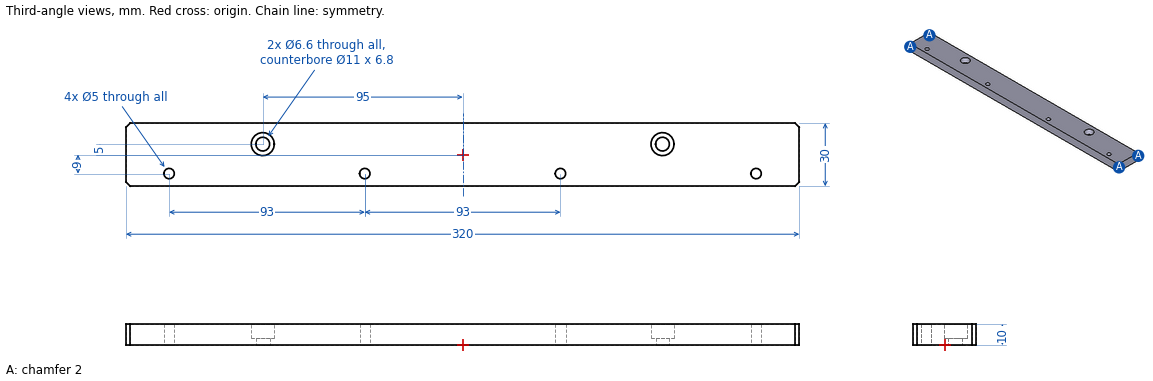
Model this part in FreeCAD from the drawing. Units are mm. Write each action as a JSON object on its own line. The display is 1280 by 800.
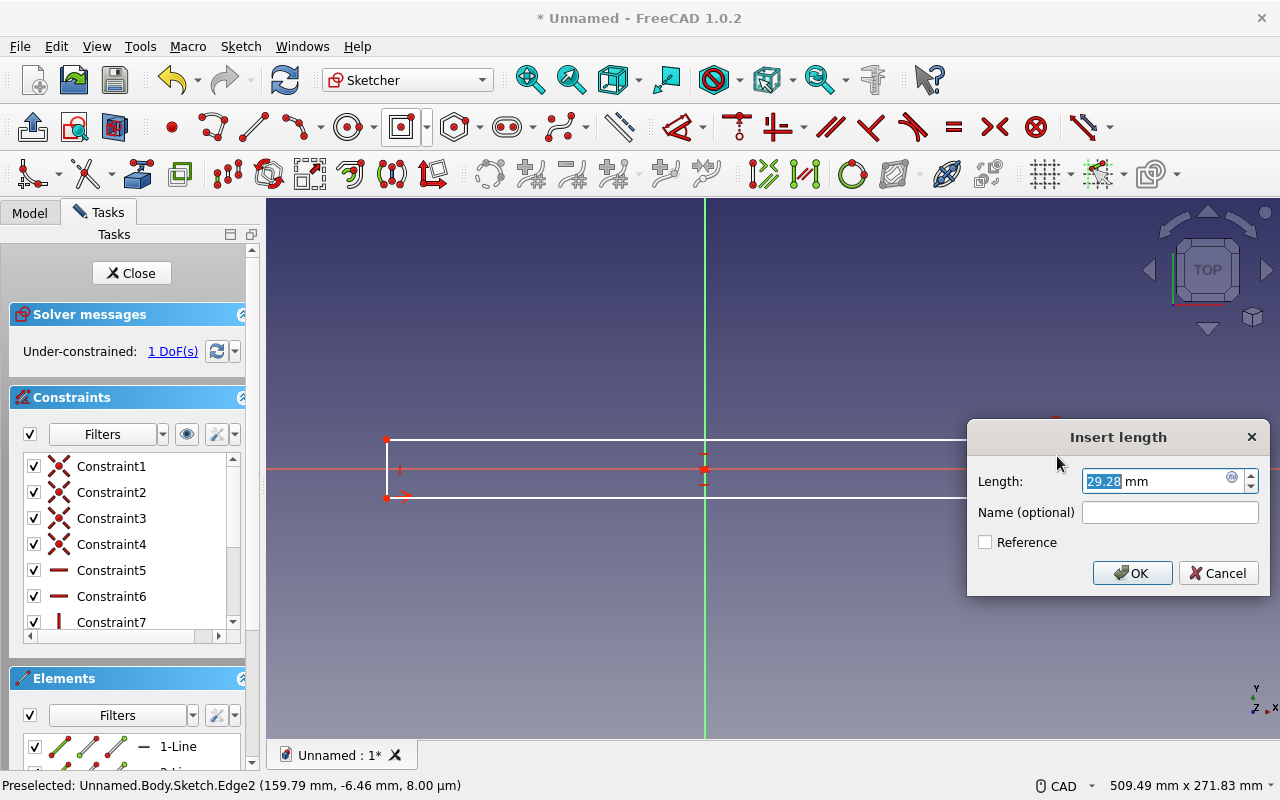
{"action": "type", "text": "30"}
{"action": "key", "text": "Return"}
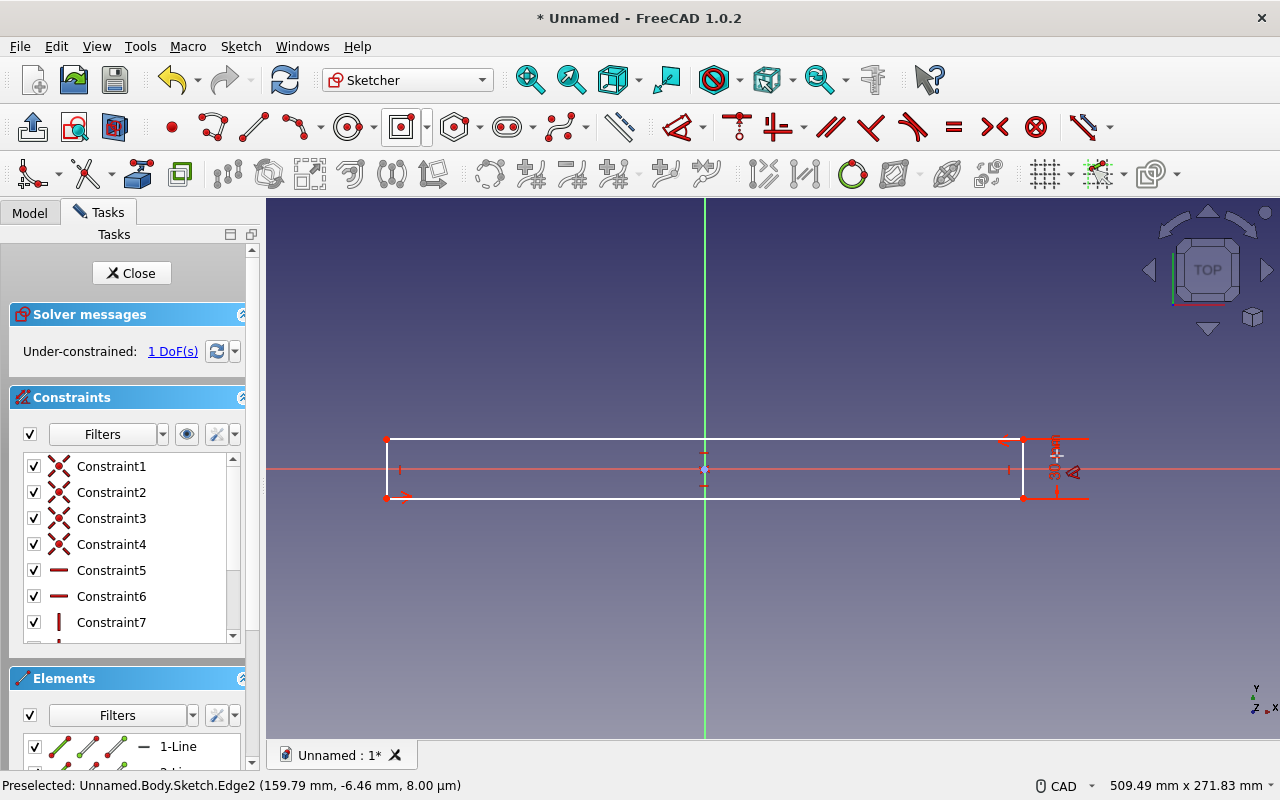
{"action": "left_click", "coordinate": [578, 499]}
{"action": "left_click", "coordinate": [559, 533]}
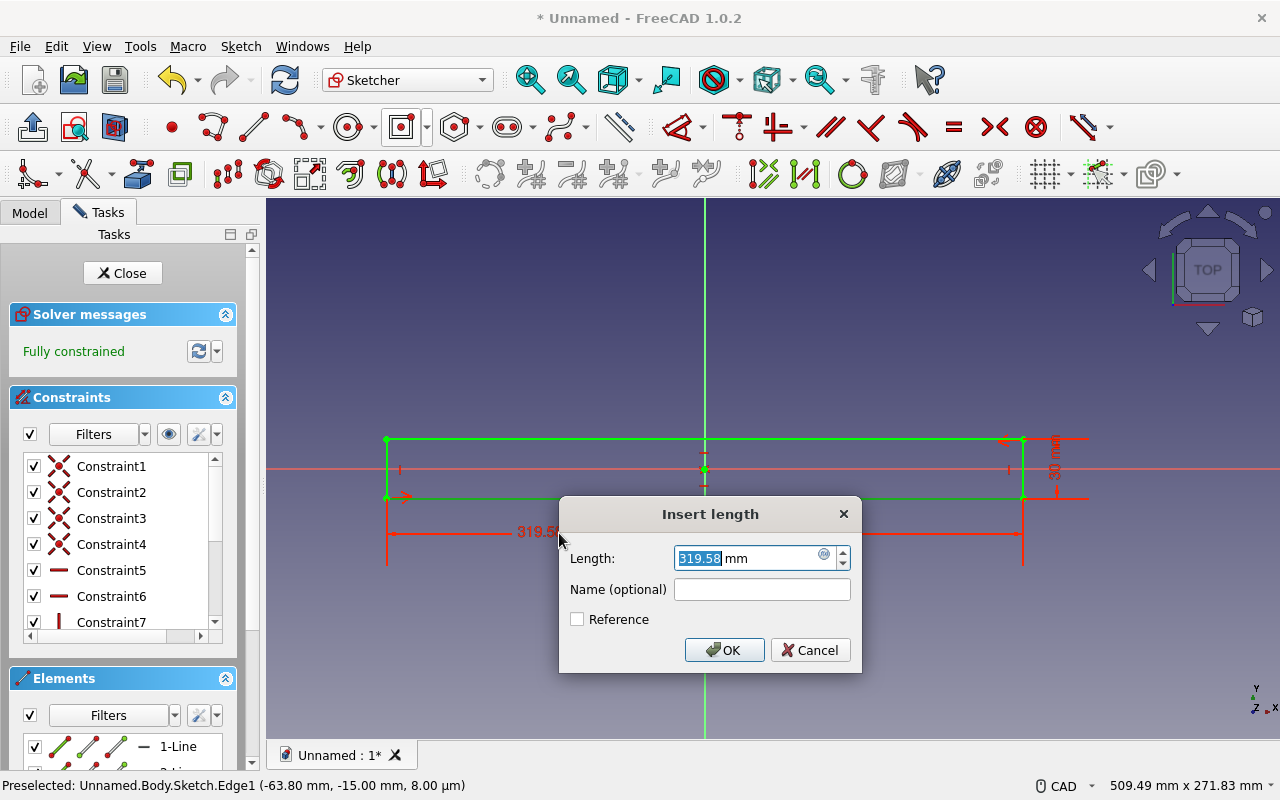
{"action": "type", "text": "320"}
{"action": "key", "text": "Return"}
{"action": "key", "text": "Escape"}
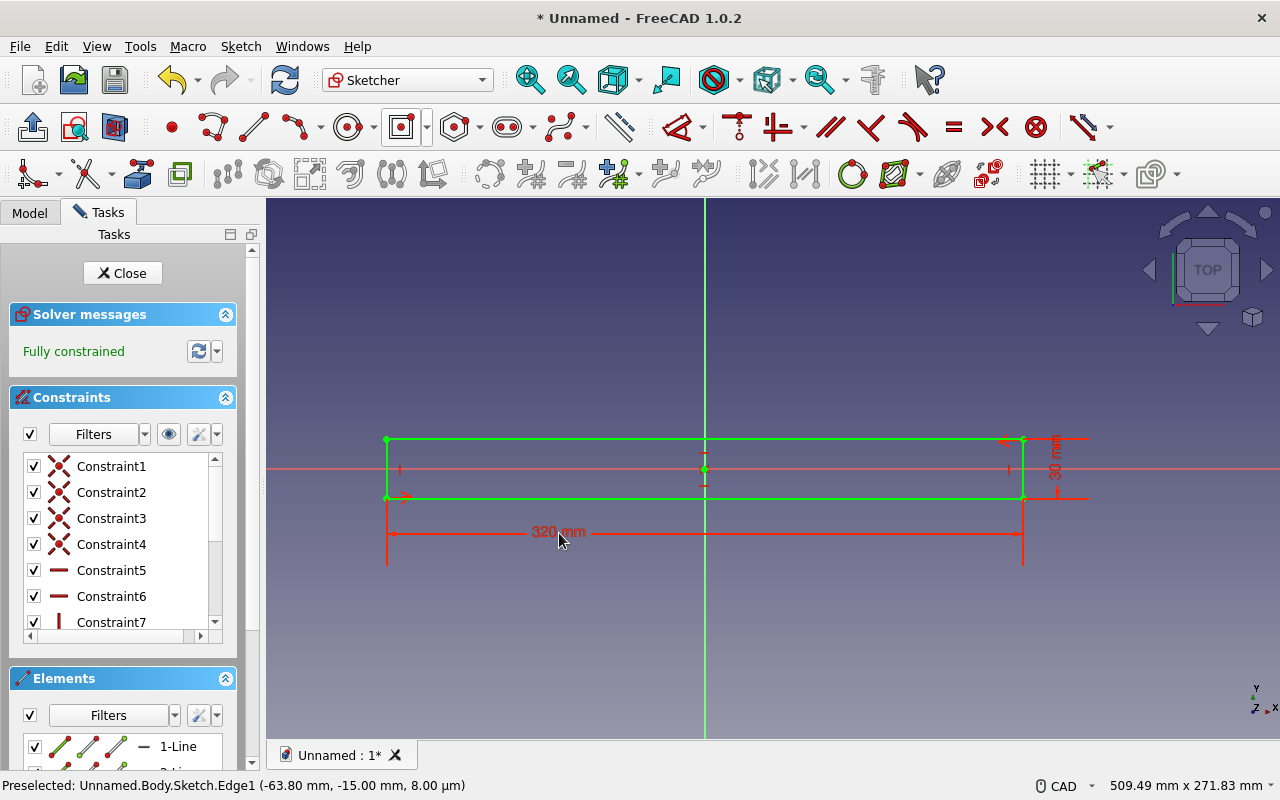
{"action": "left_click", "coordinate": [123, 273]}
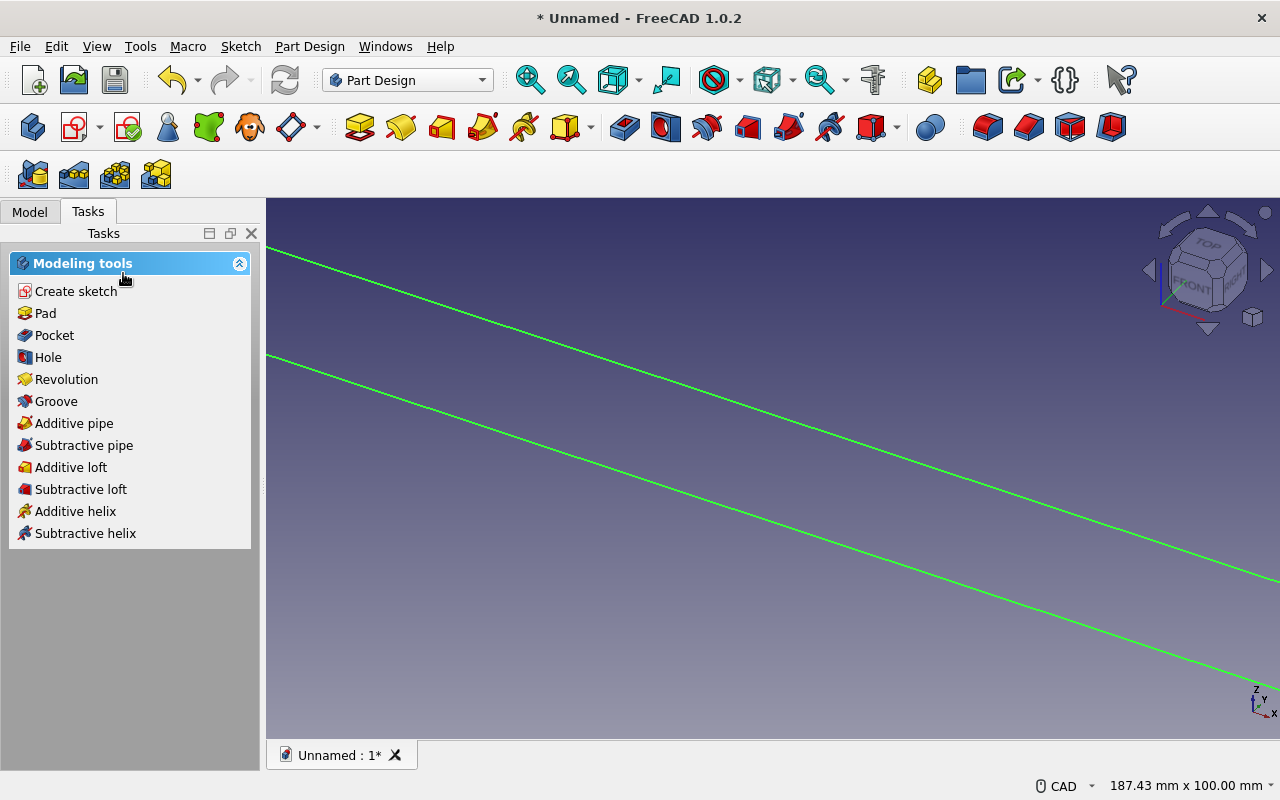
{"action": "left_click", "coordinate": [360, 128]}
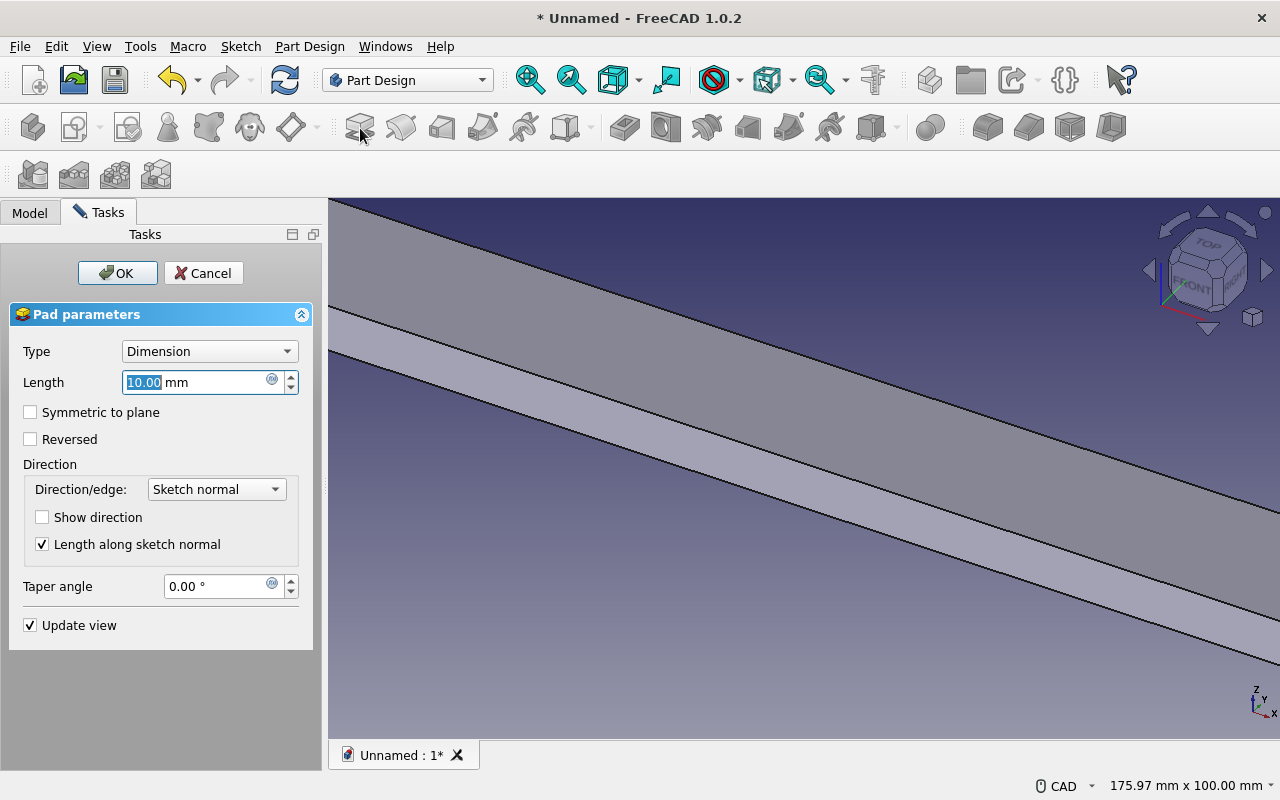
{"action": "type", "text": "10"}
{"action": "key", "text": "Tab"}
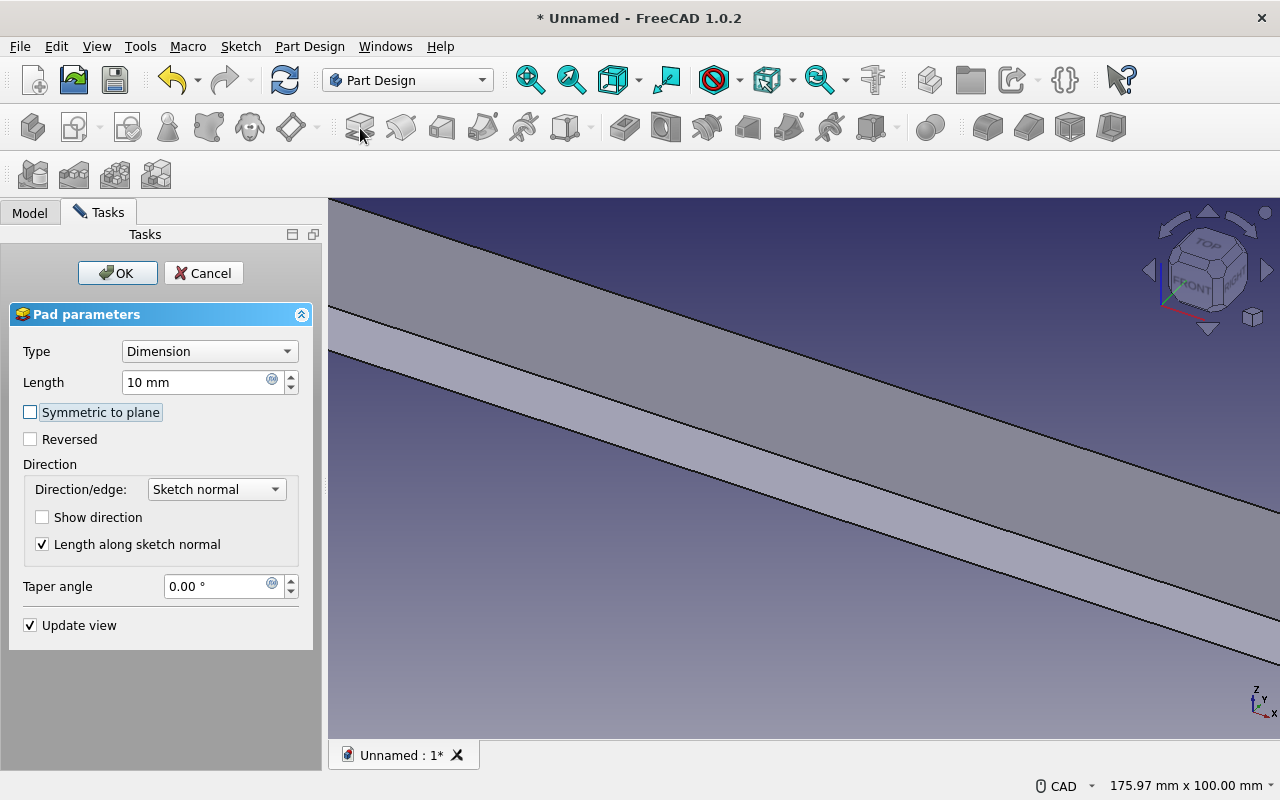
{"action": "left_click", "coordinate": [118, 273]}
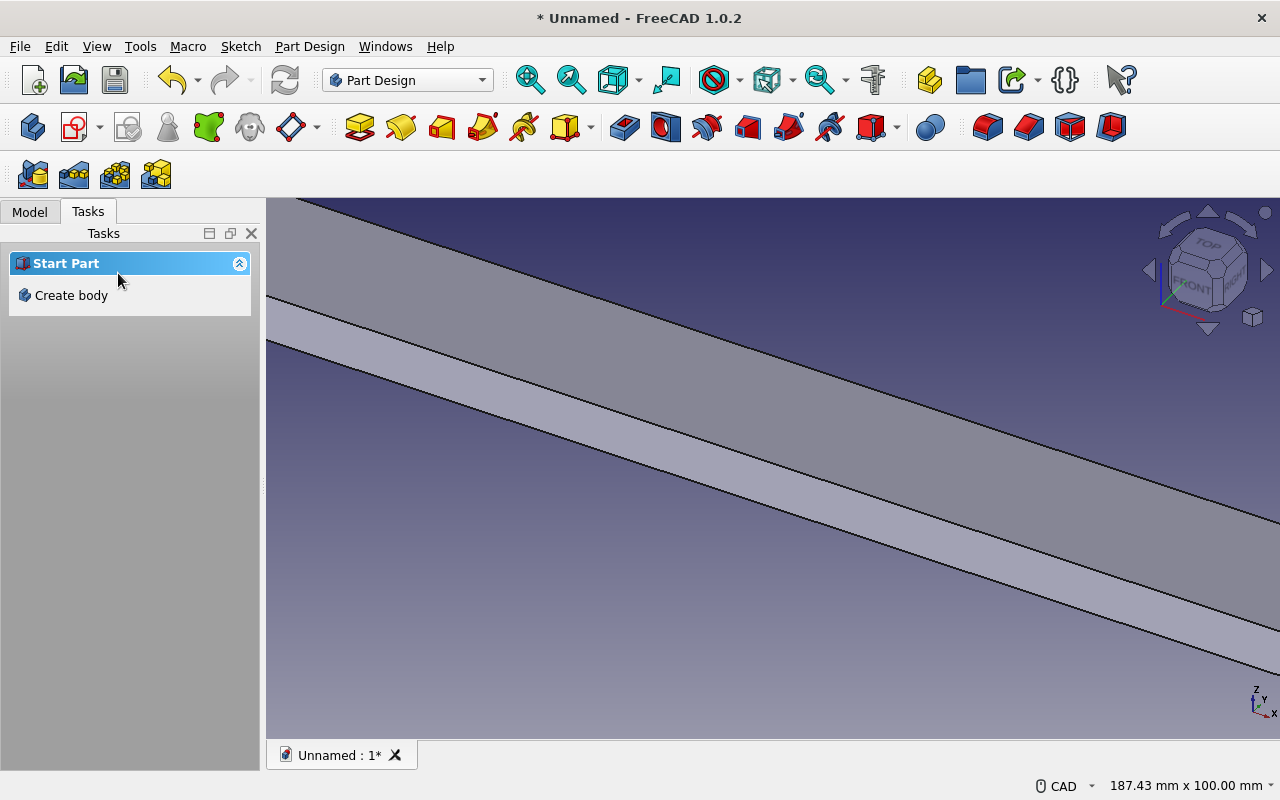
{"action": "left_click", "coordinate": [531, 80]}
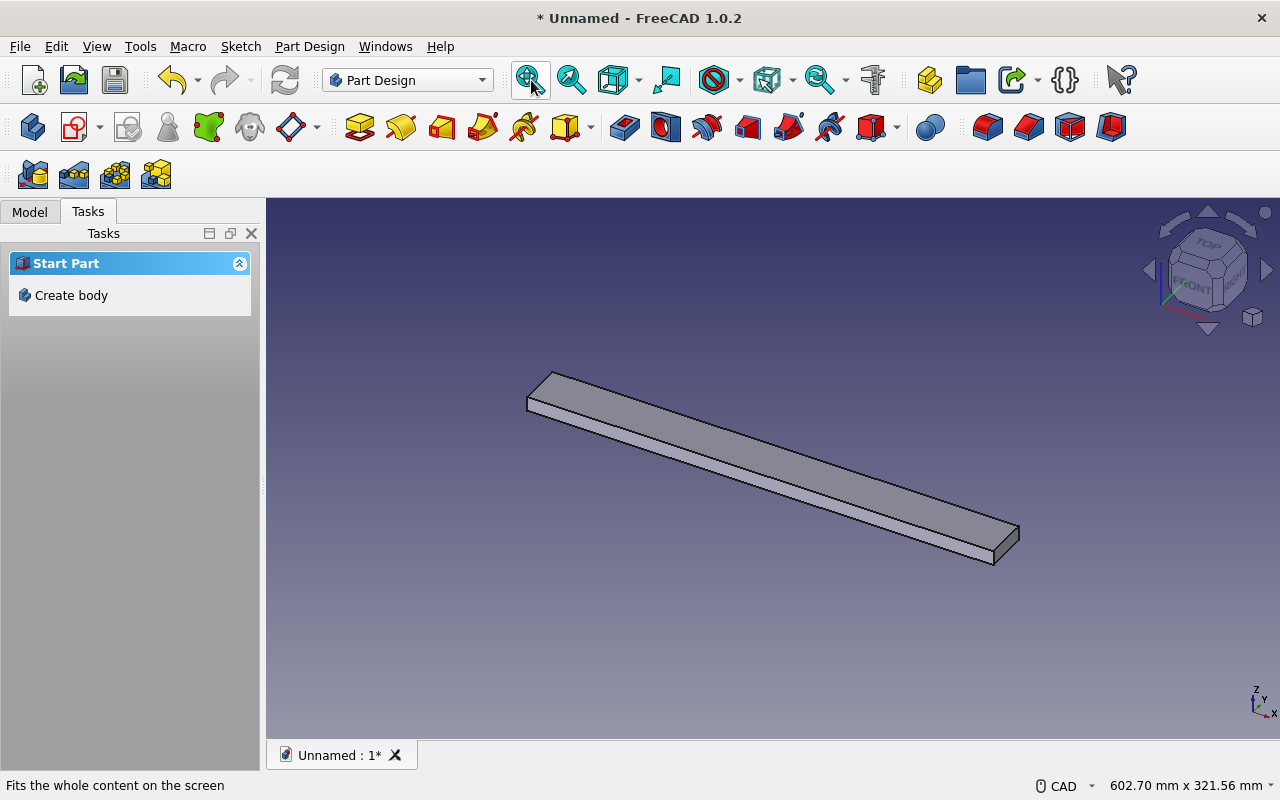
{"action": "left_click", "coordinate": [994, 557]}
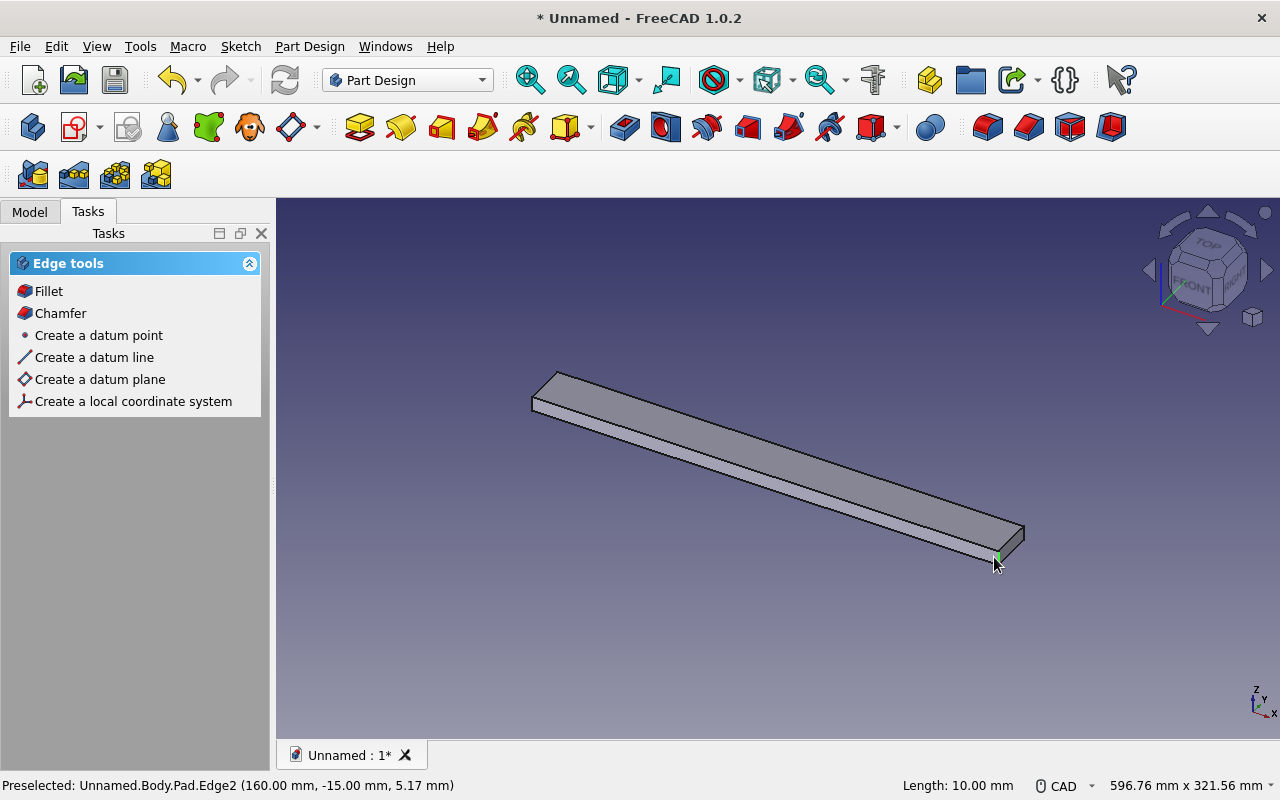
{"action": "scroll", "coordinate": [532, 403], "scroll_direction": "up", "scroll_amount": 5}